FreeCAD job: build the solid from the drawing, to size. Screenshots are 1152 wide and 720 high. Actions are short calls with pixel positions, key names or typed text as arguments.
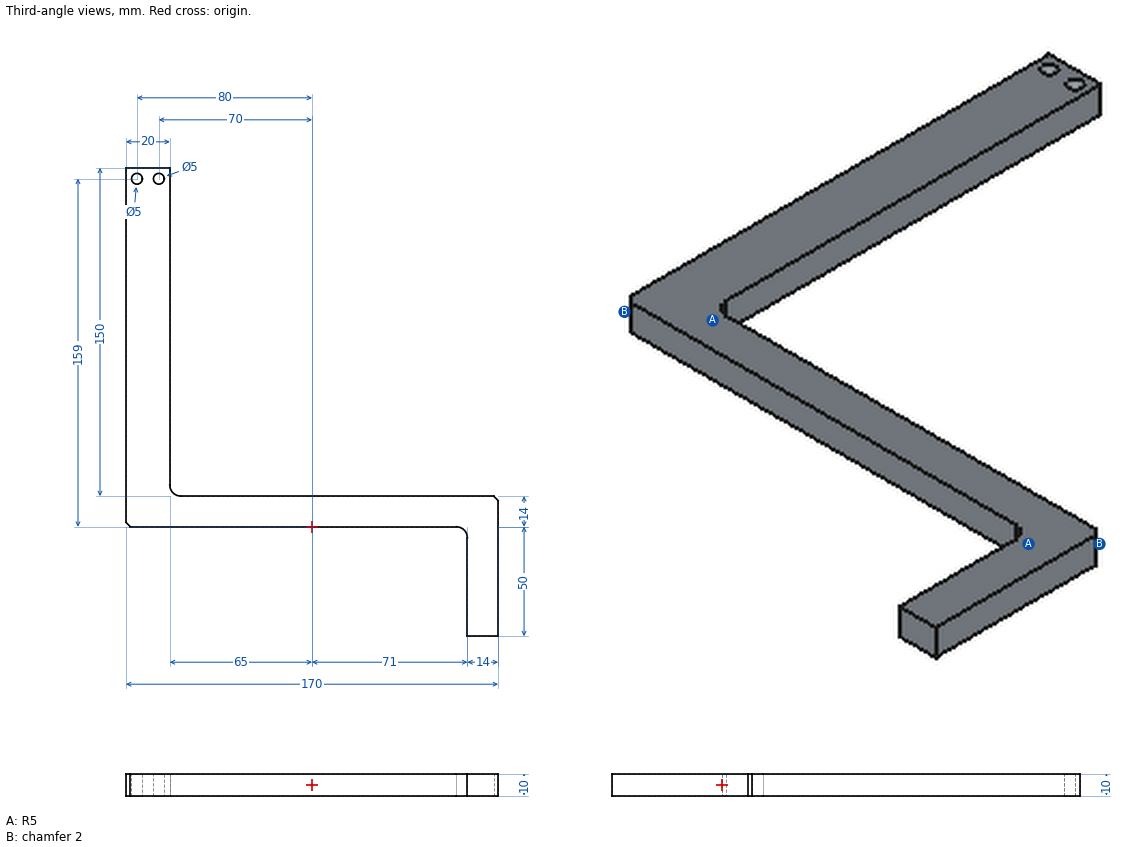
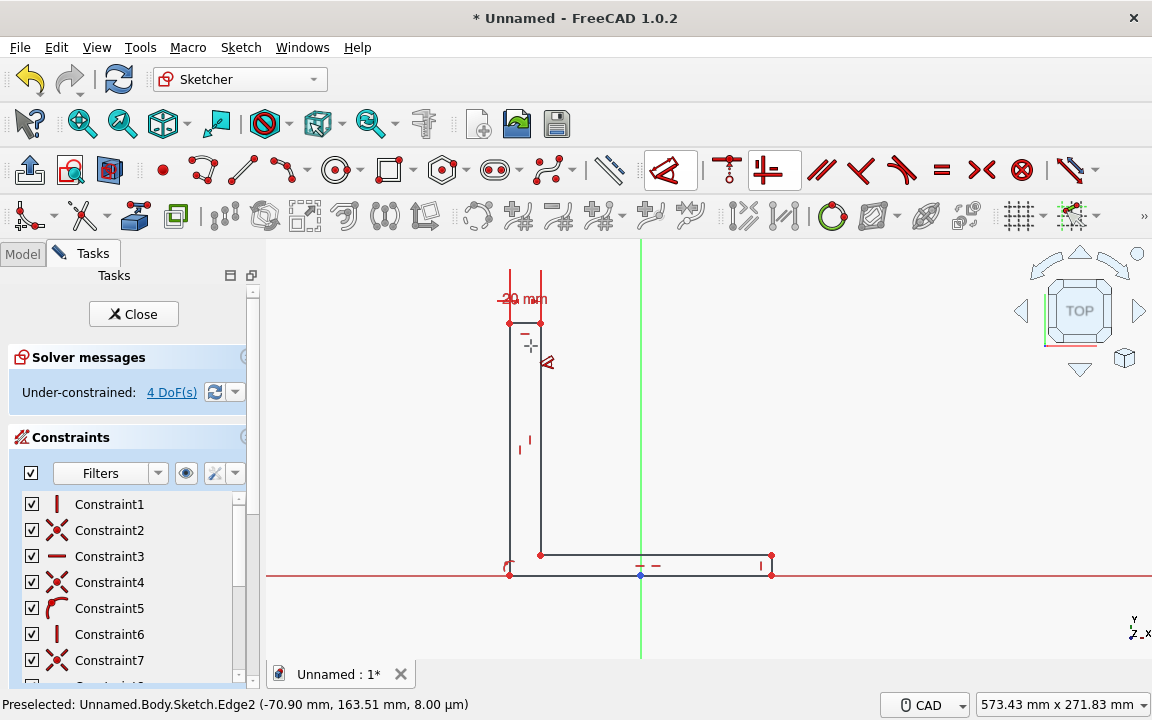
scroll(772, 570, up, 5)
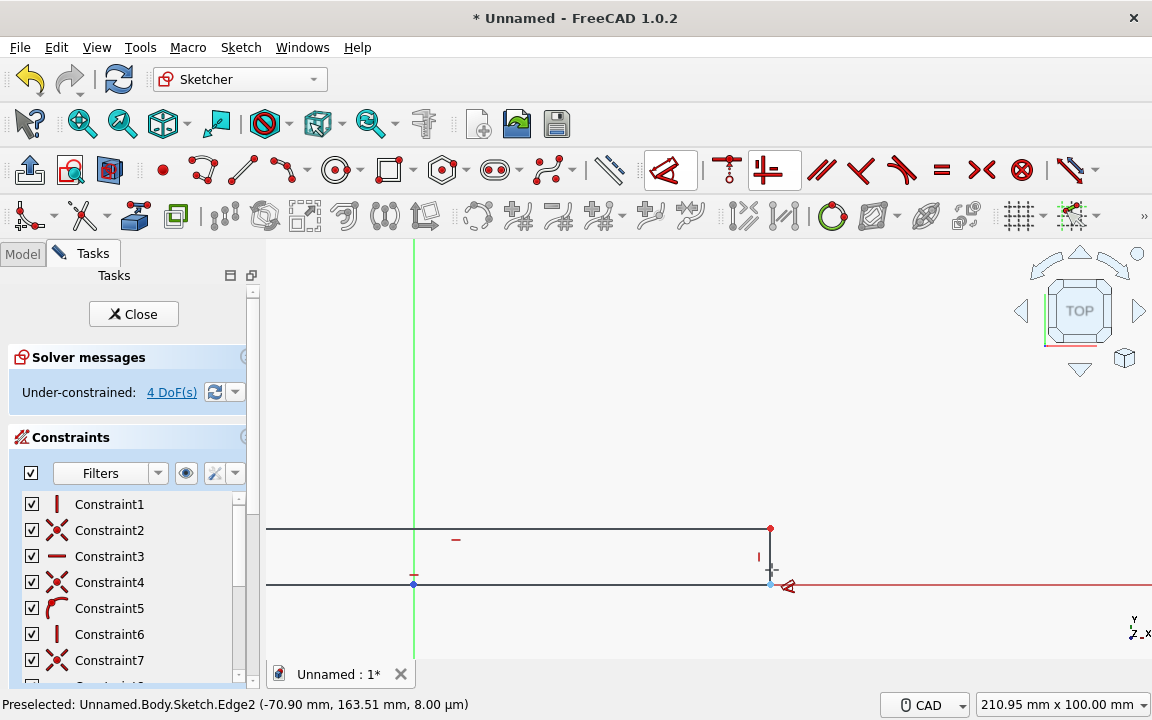
click(770, 568)
click(804, 557)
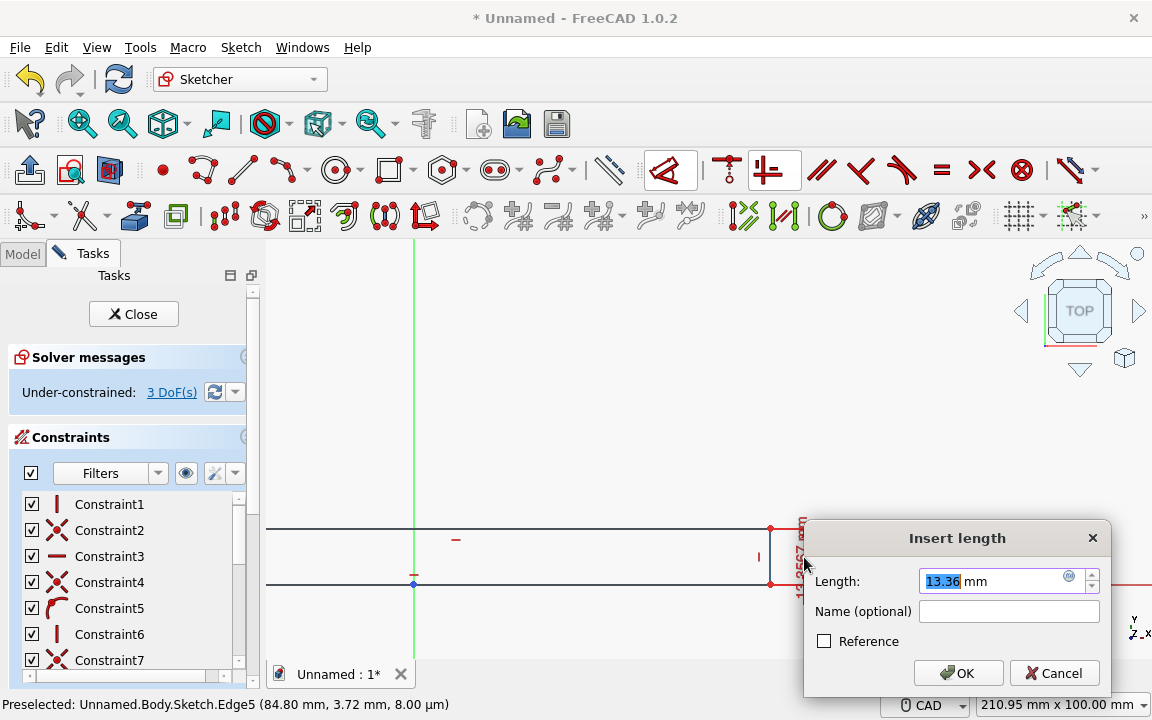
text(14)
key(Return)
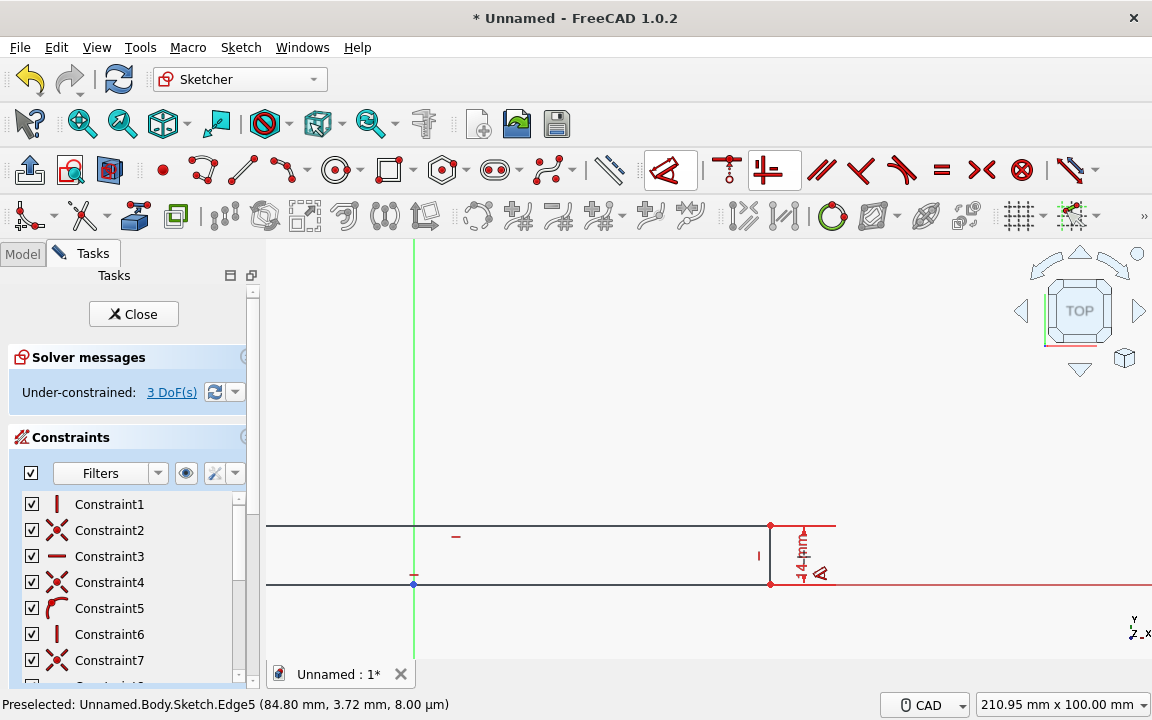
scroll(772, 571, down, 5)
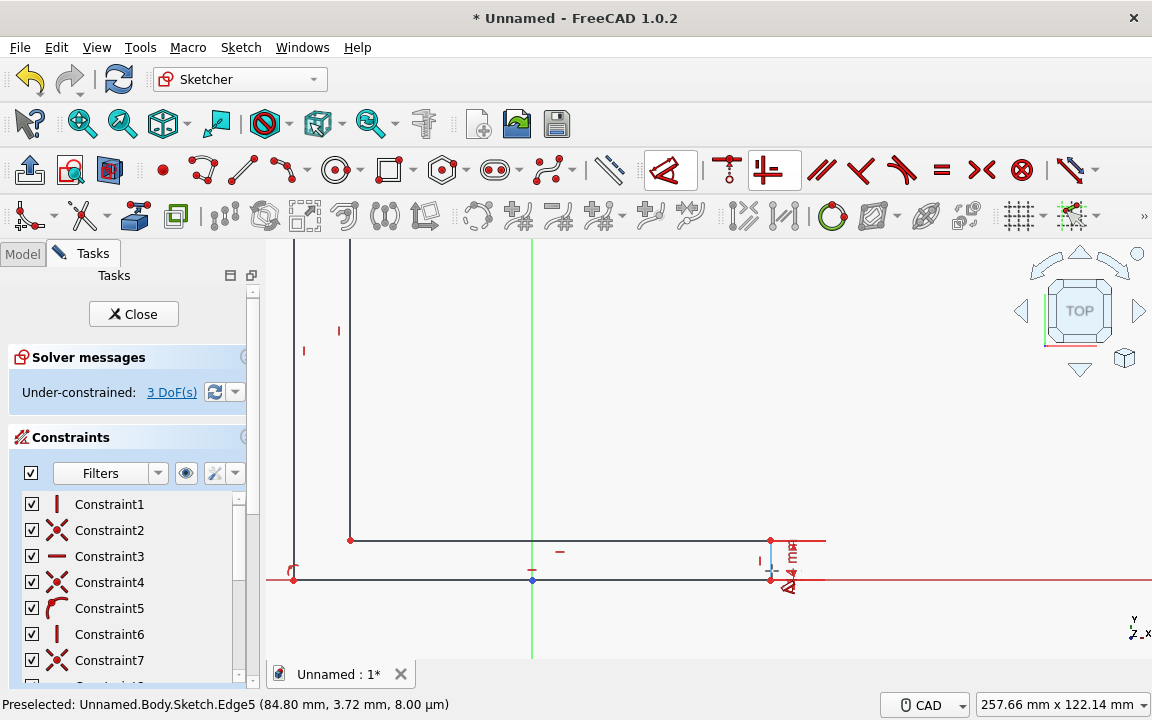
click(541, 486)
click(575, 439)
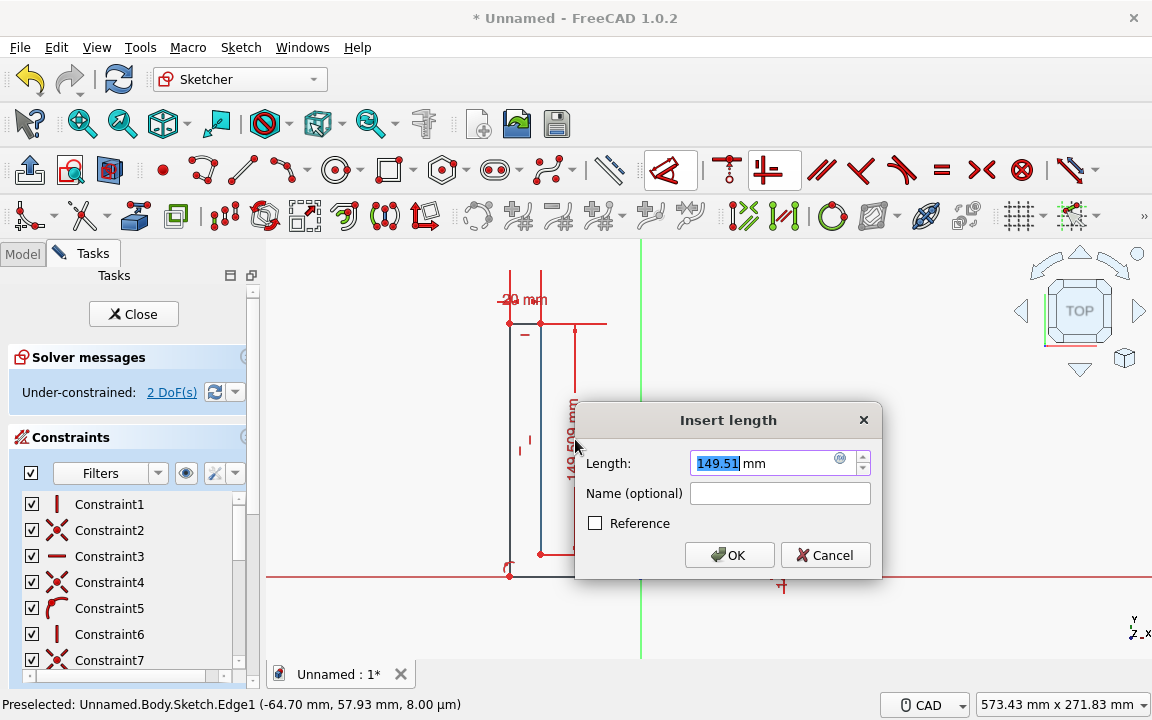
text(150)
key(Return)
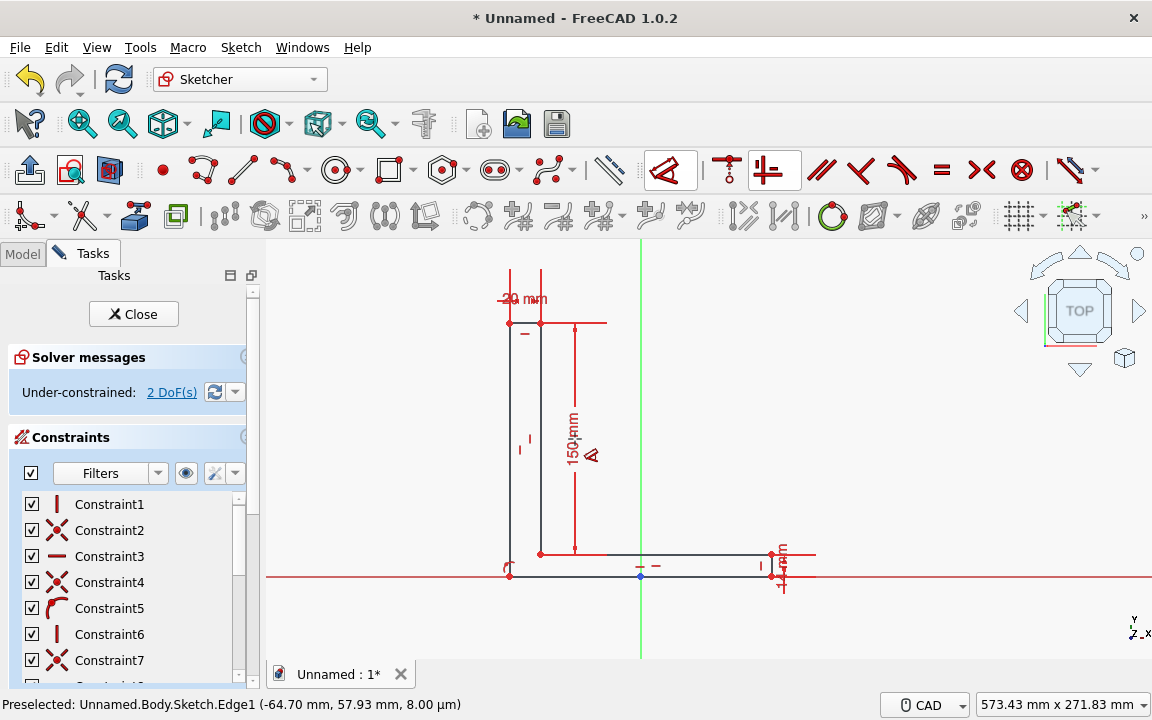
click(588, 577)
click(580, 611)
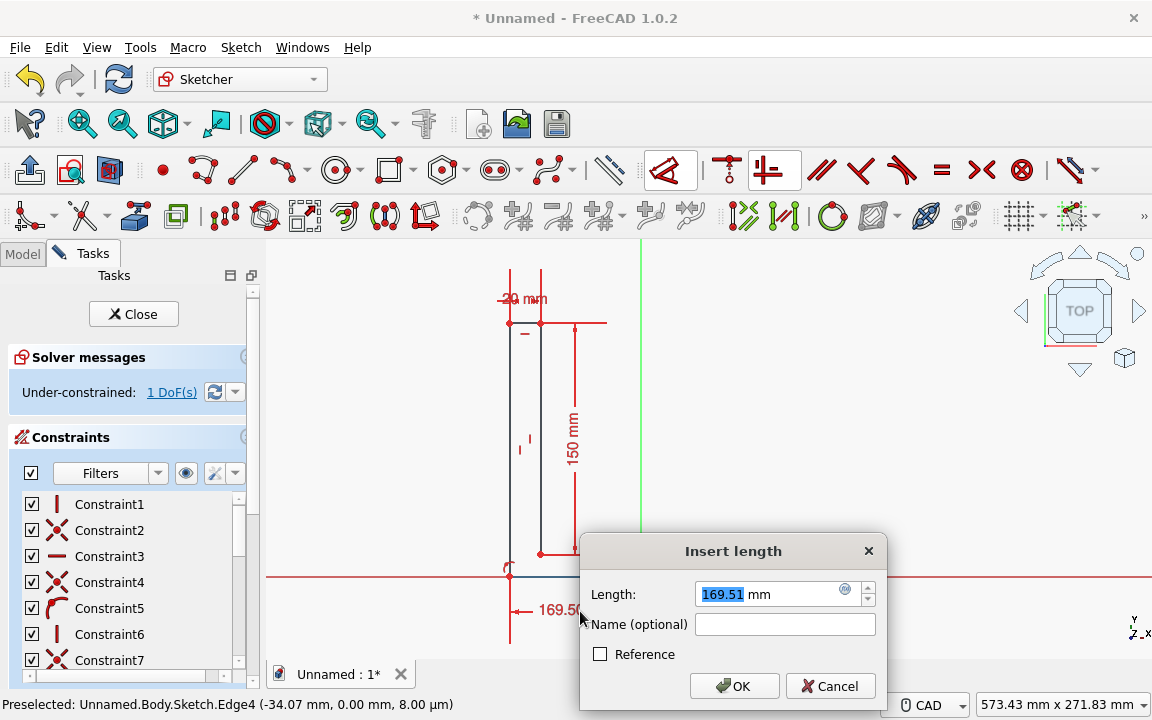
text(170)
key(Return)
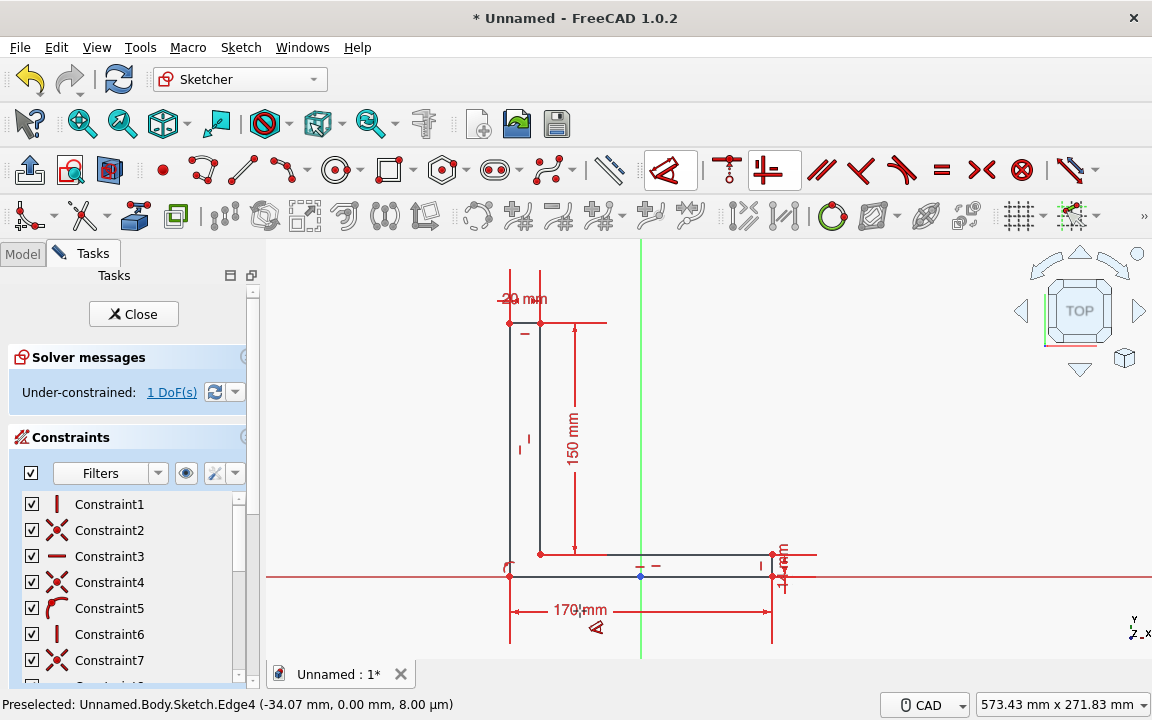
click(540, 555)
click(591, 521)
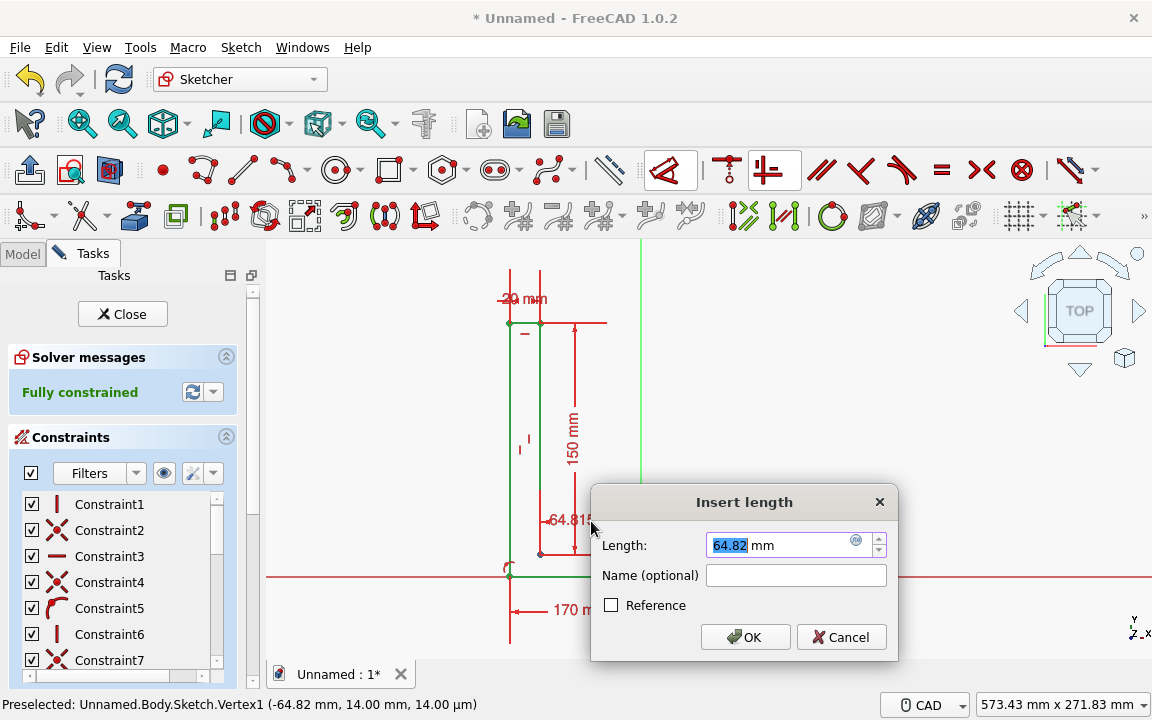
text(65)
key(Return)
key(Escape)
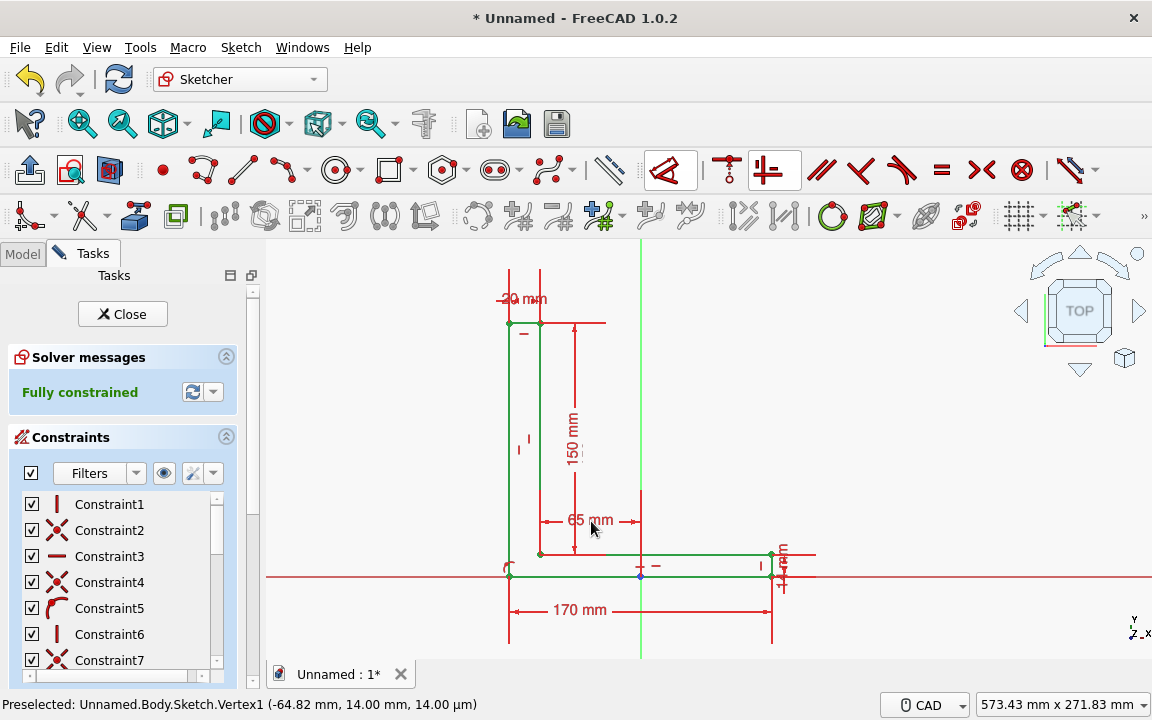
click(123, 314)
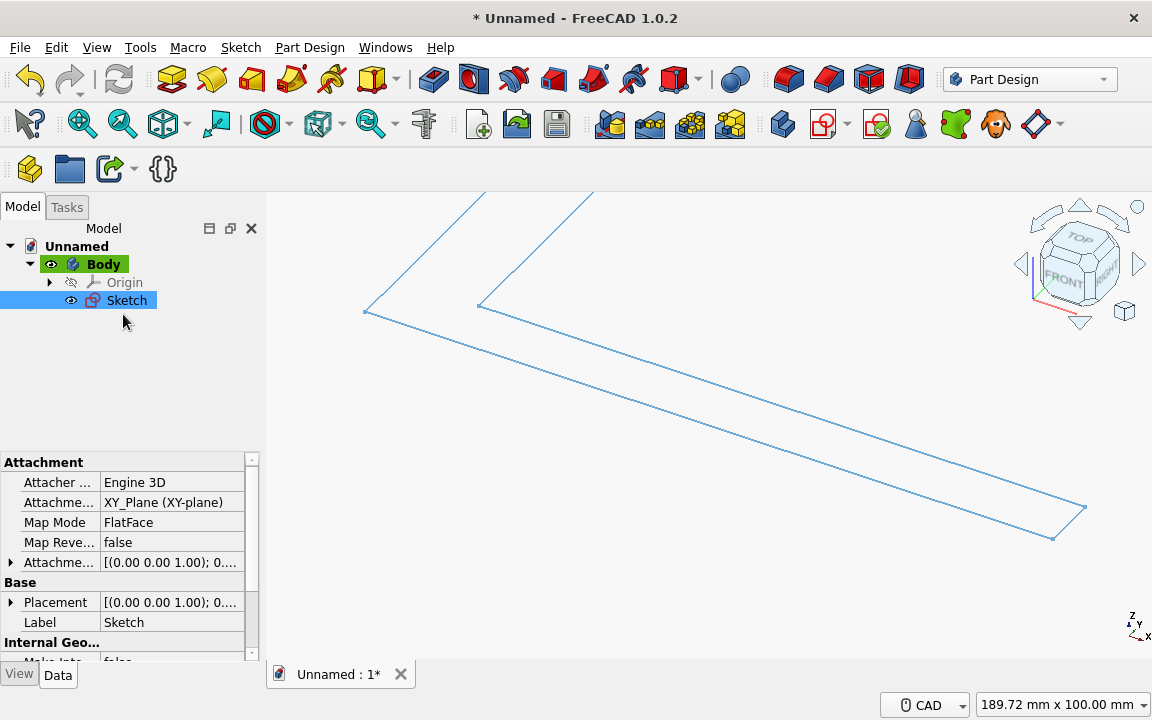
click(172, 80)